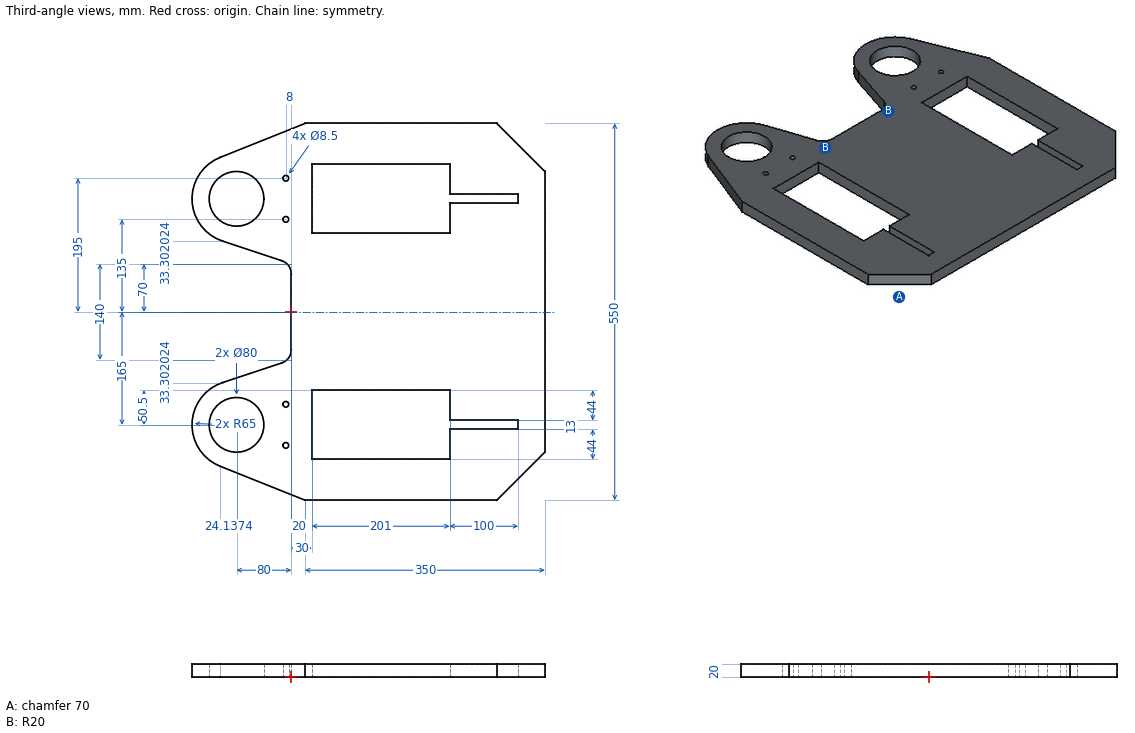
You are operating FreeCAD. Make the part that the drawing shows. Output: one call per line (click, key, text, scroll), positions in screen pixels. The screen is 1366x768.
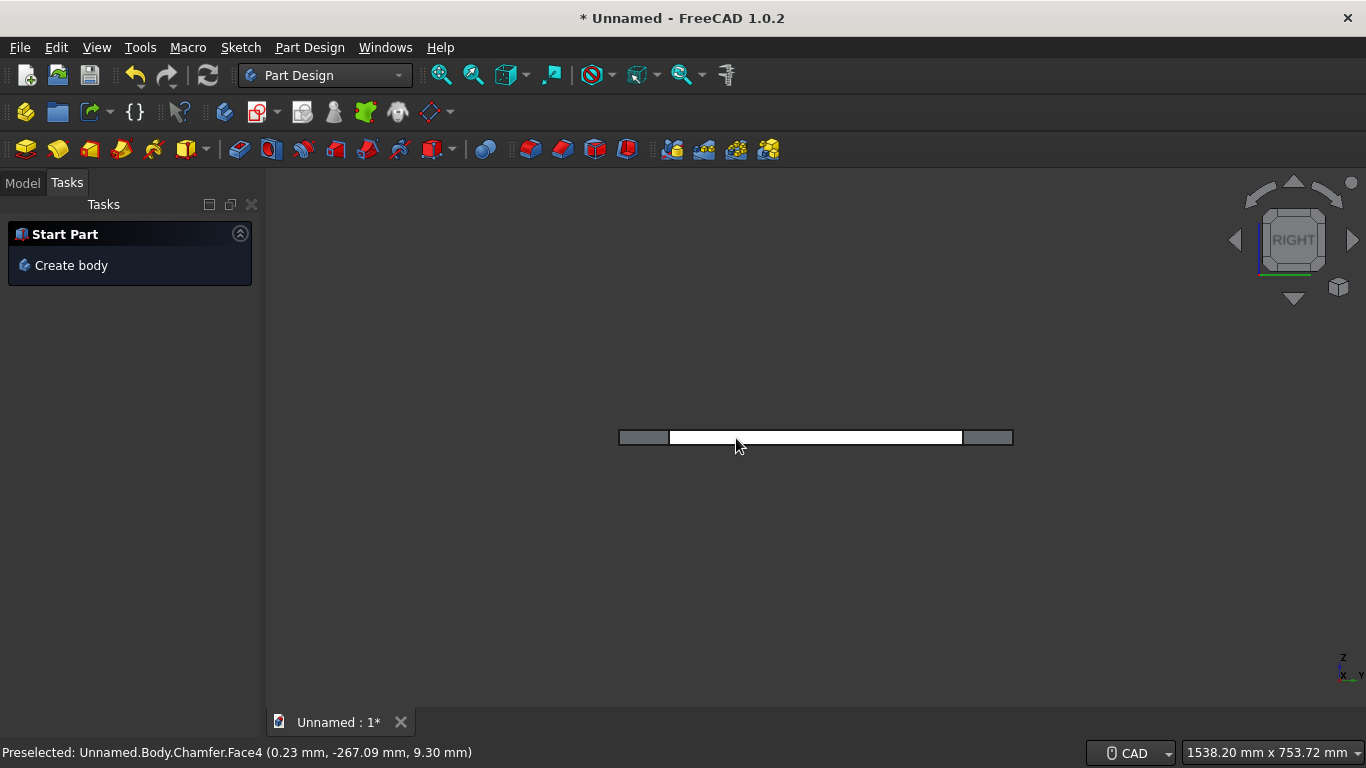
key(v)
key(f)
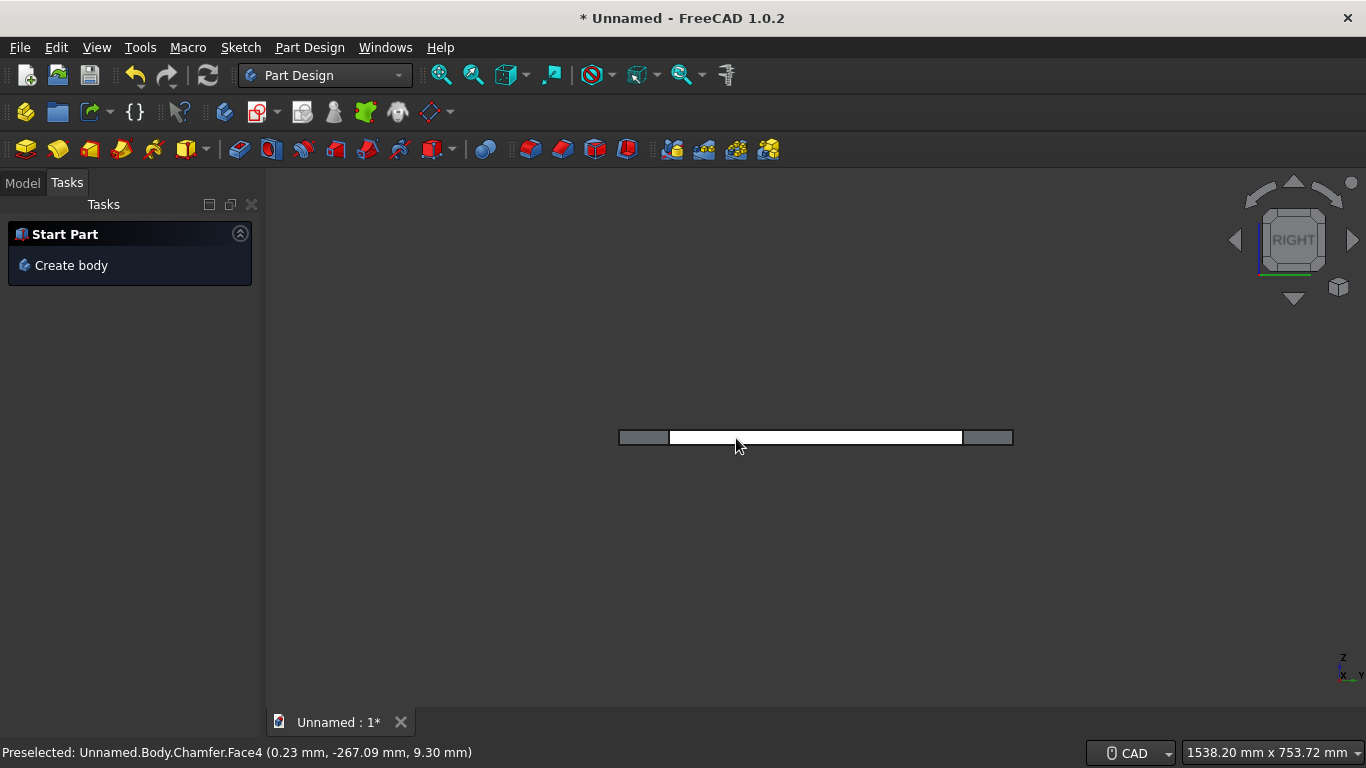
scroll(766, 436, up, 6)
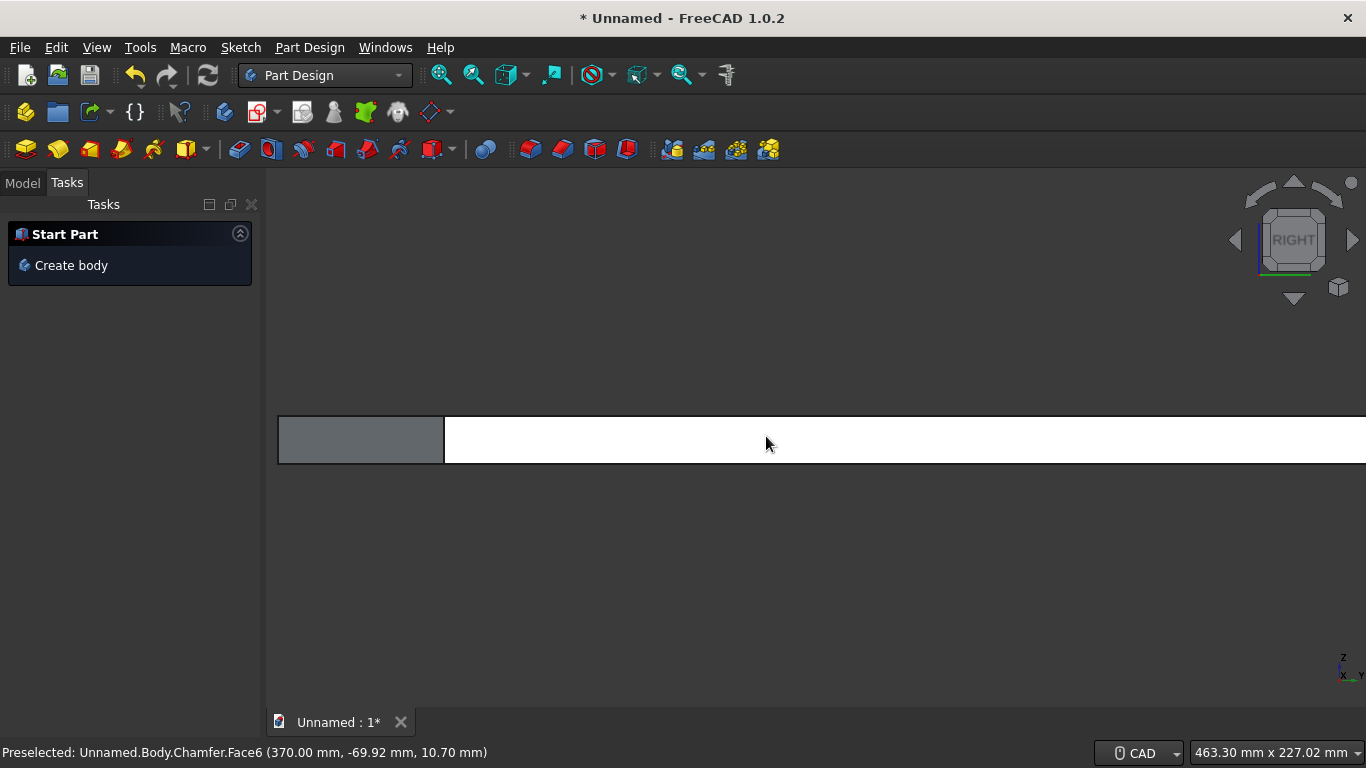
key(v)
key(f)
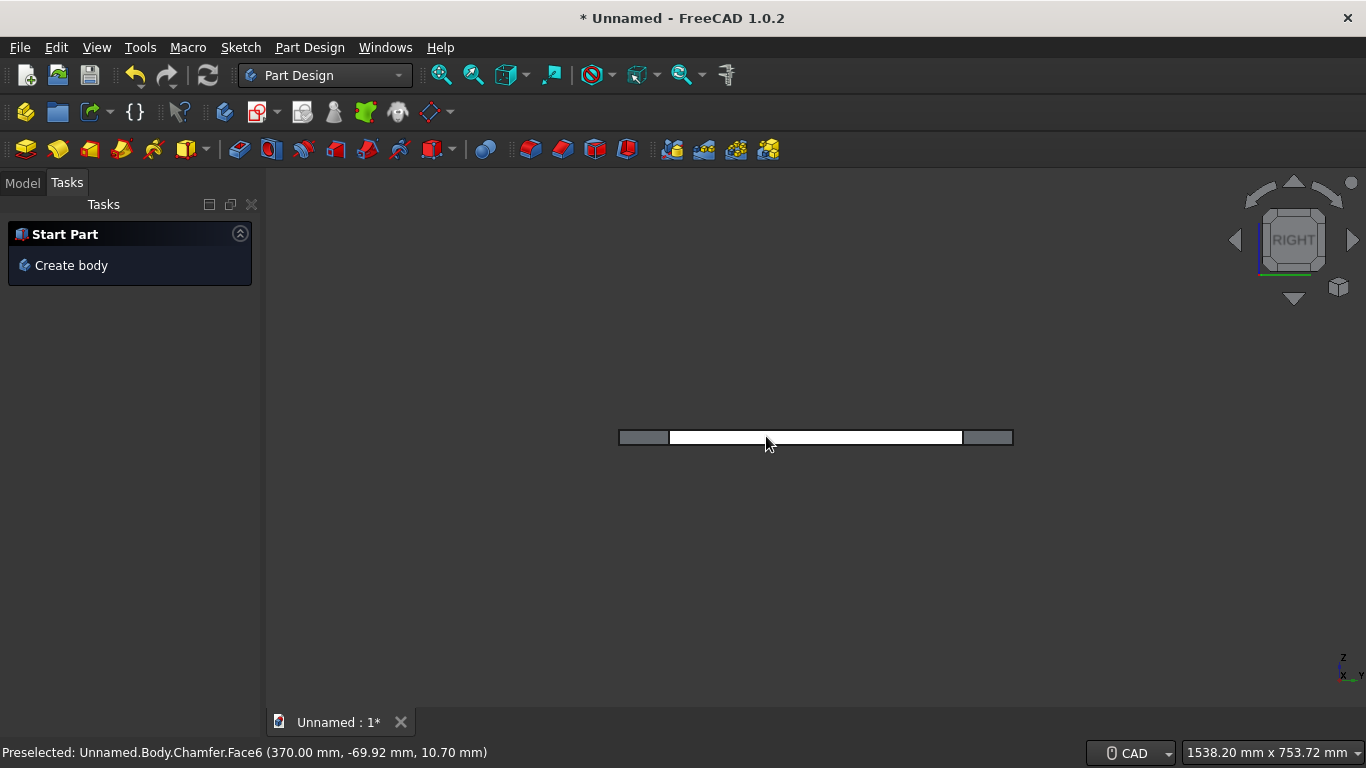
key(5)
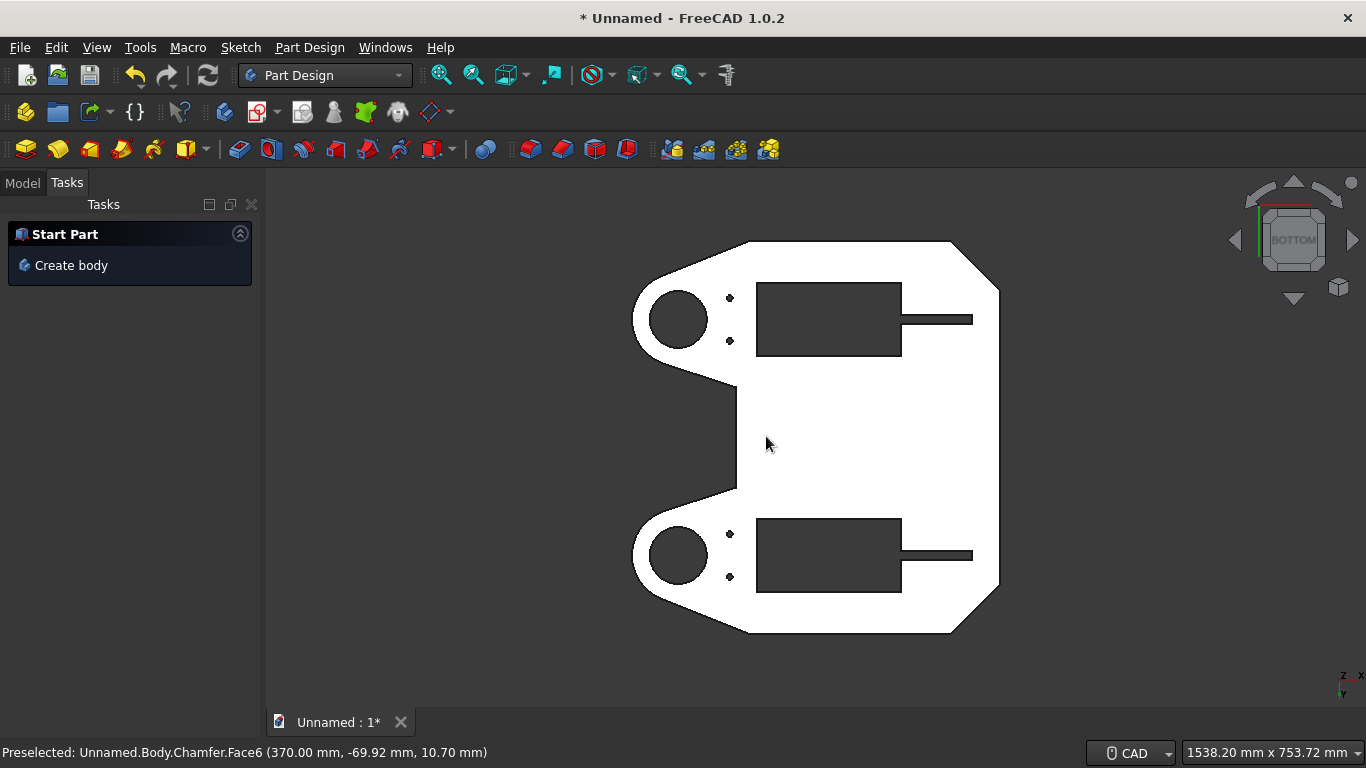
scroll(736, 386, up, 6)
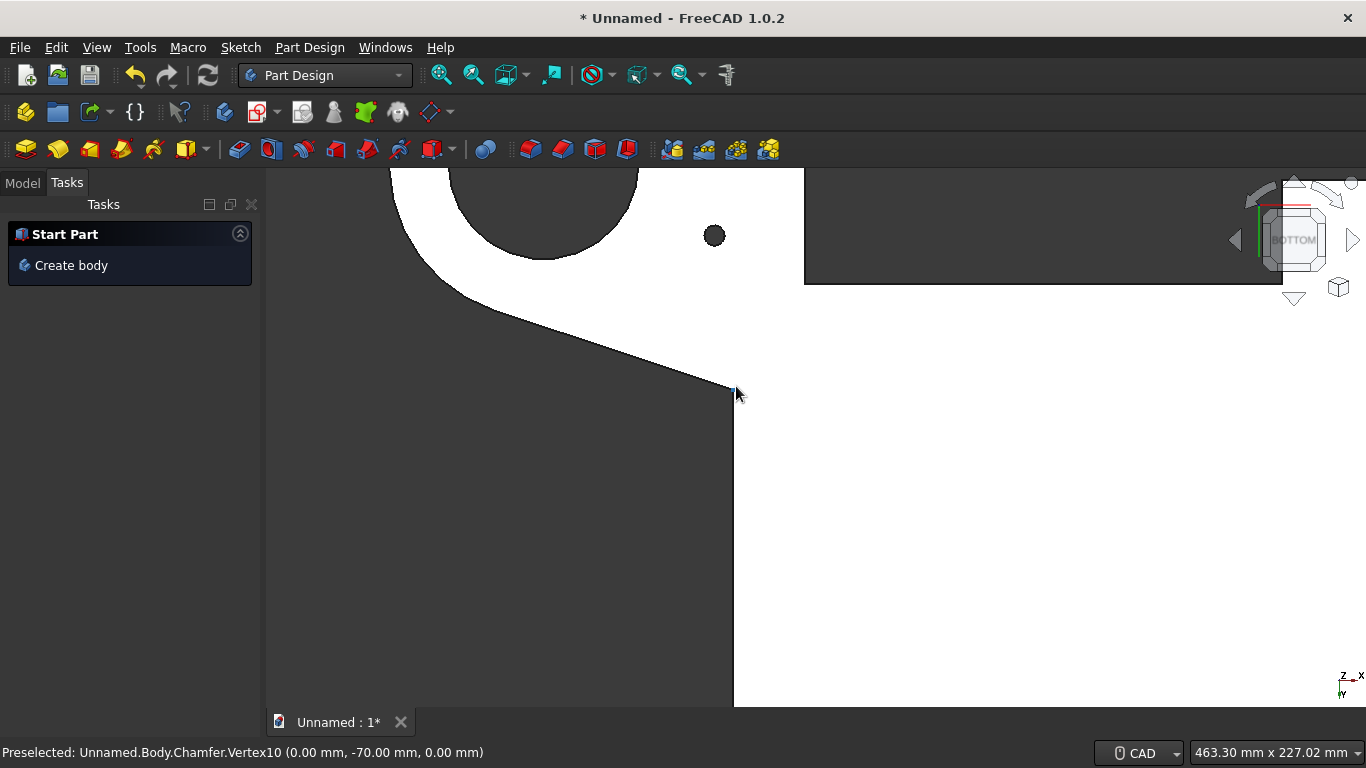
key(v)
key(f)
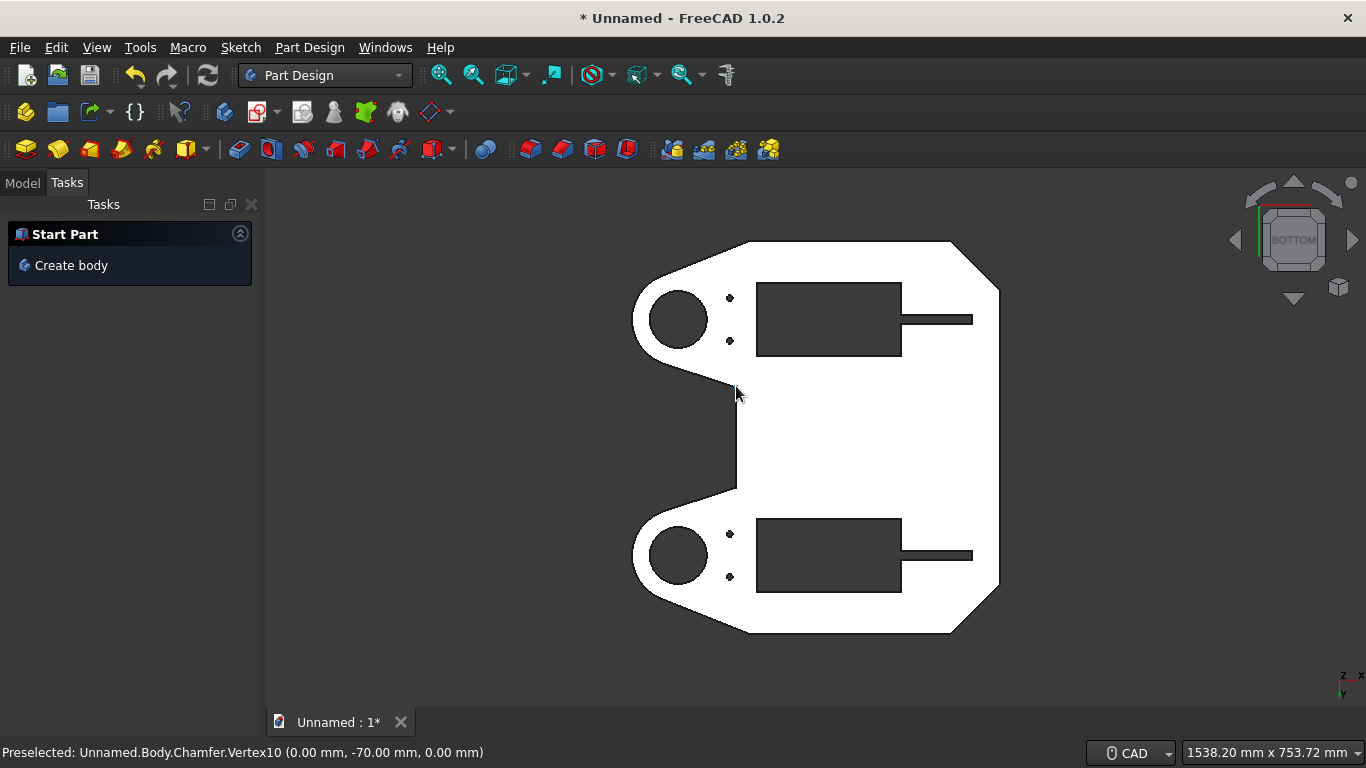
key(4)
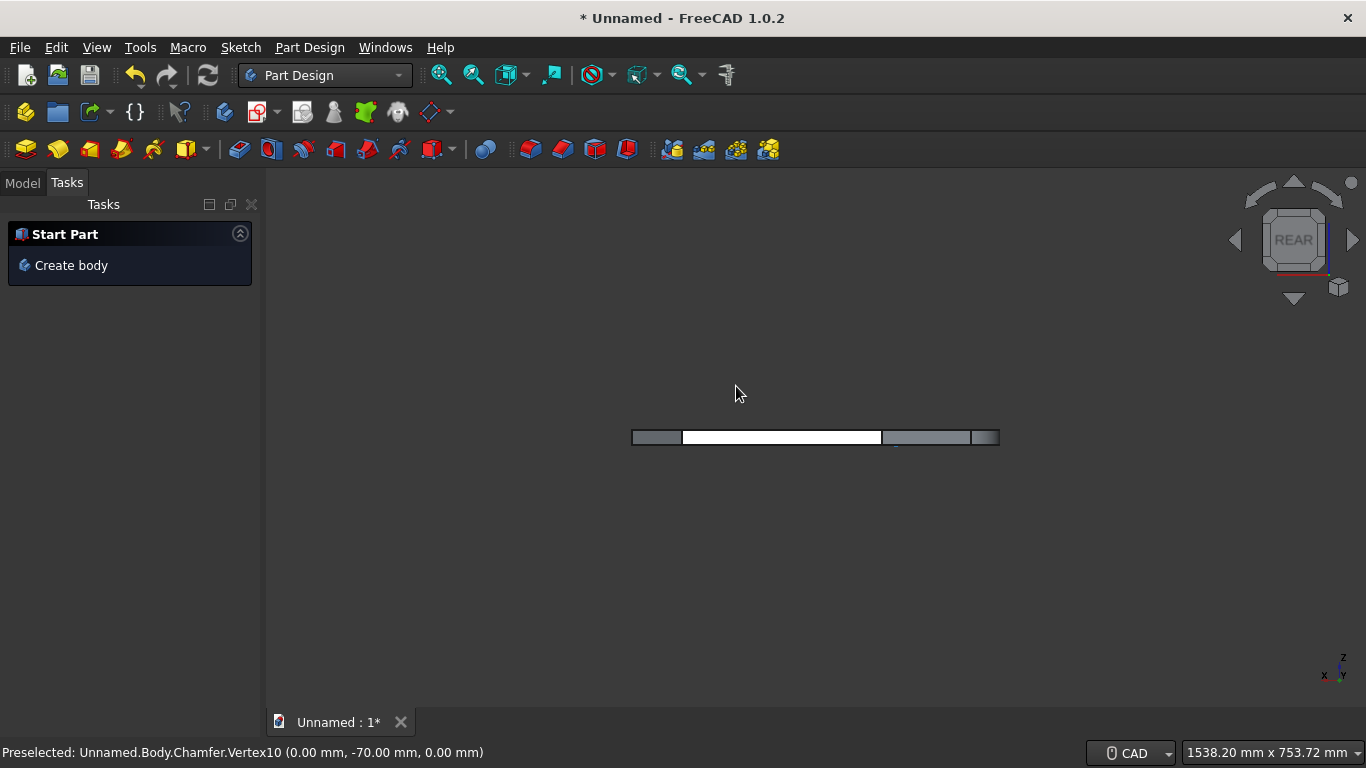
click(442, 76)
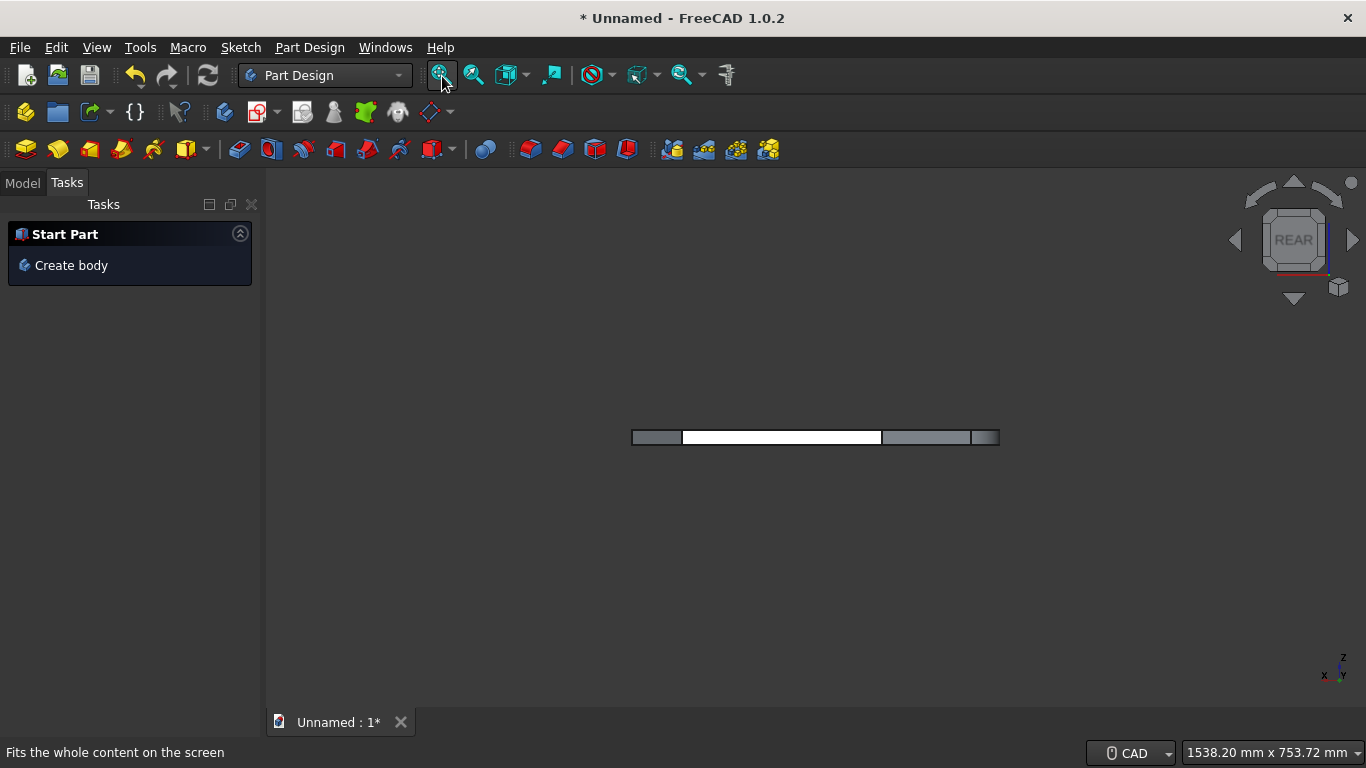
scroll(896, 437, up, 6)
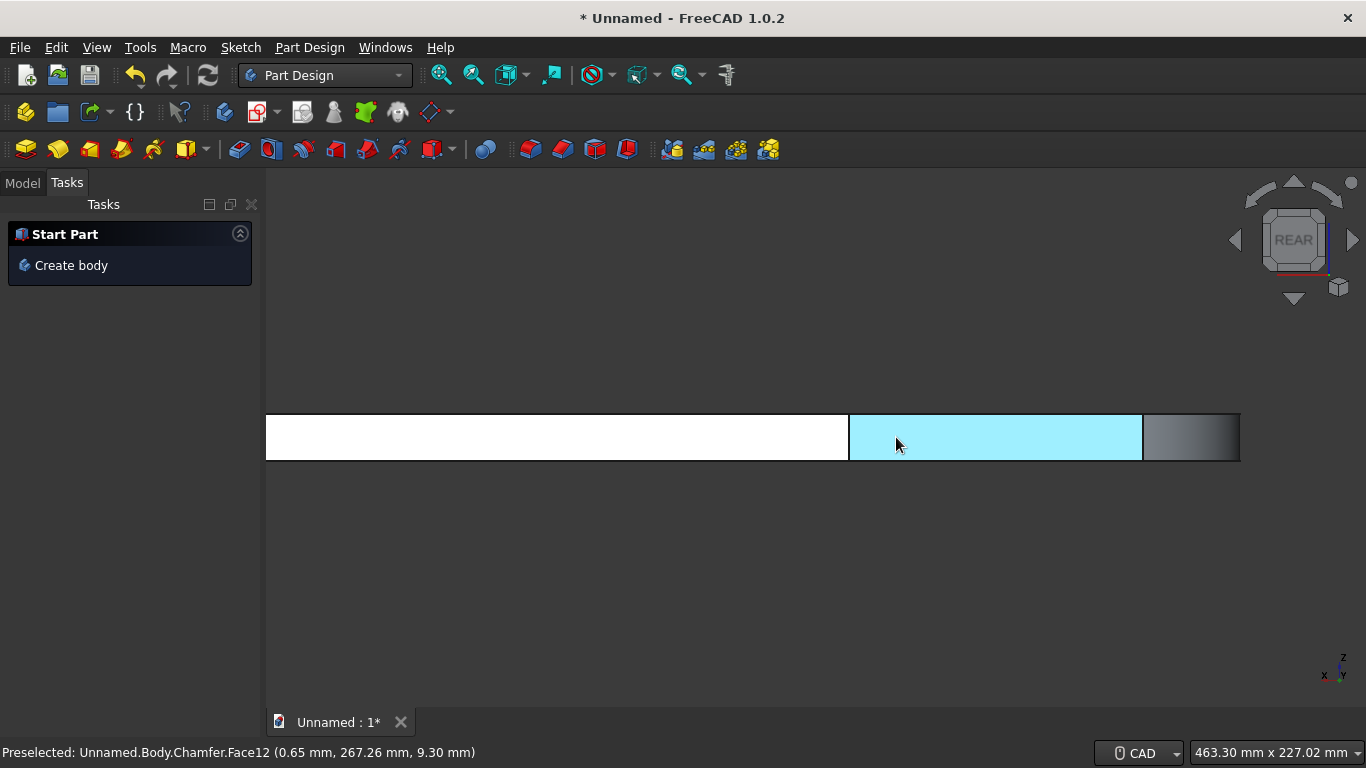
click(442, 76)